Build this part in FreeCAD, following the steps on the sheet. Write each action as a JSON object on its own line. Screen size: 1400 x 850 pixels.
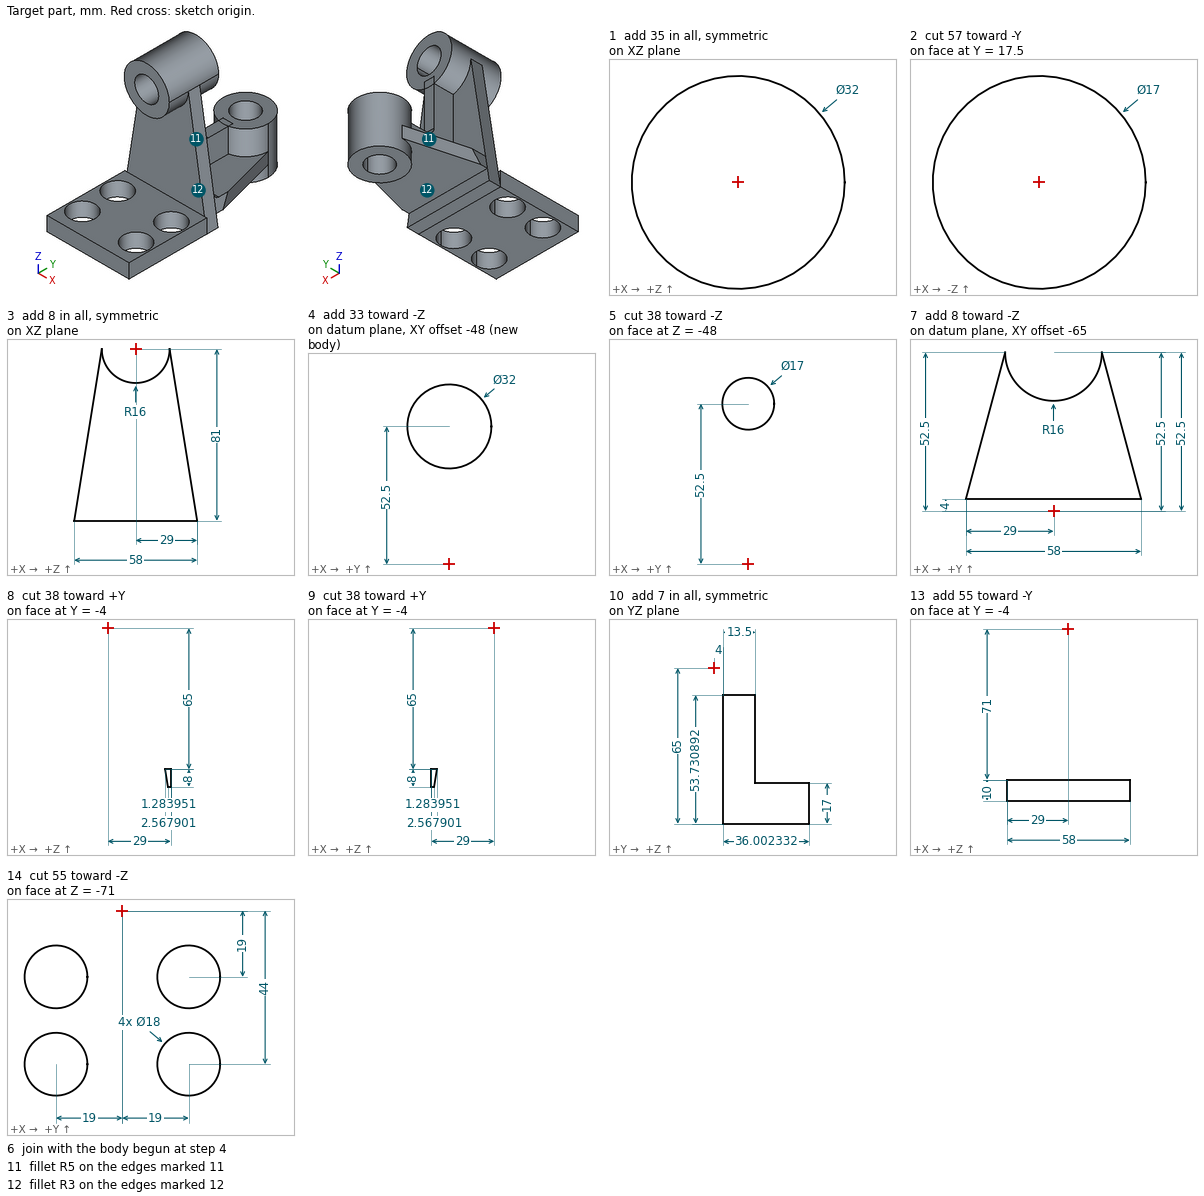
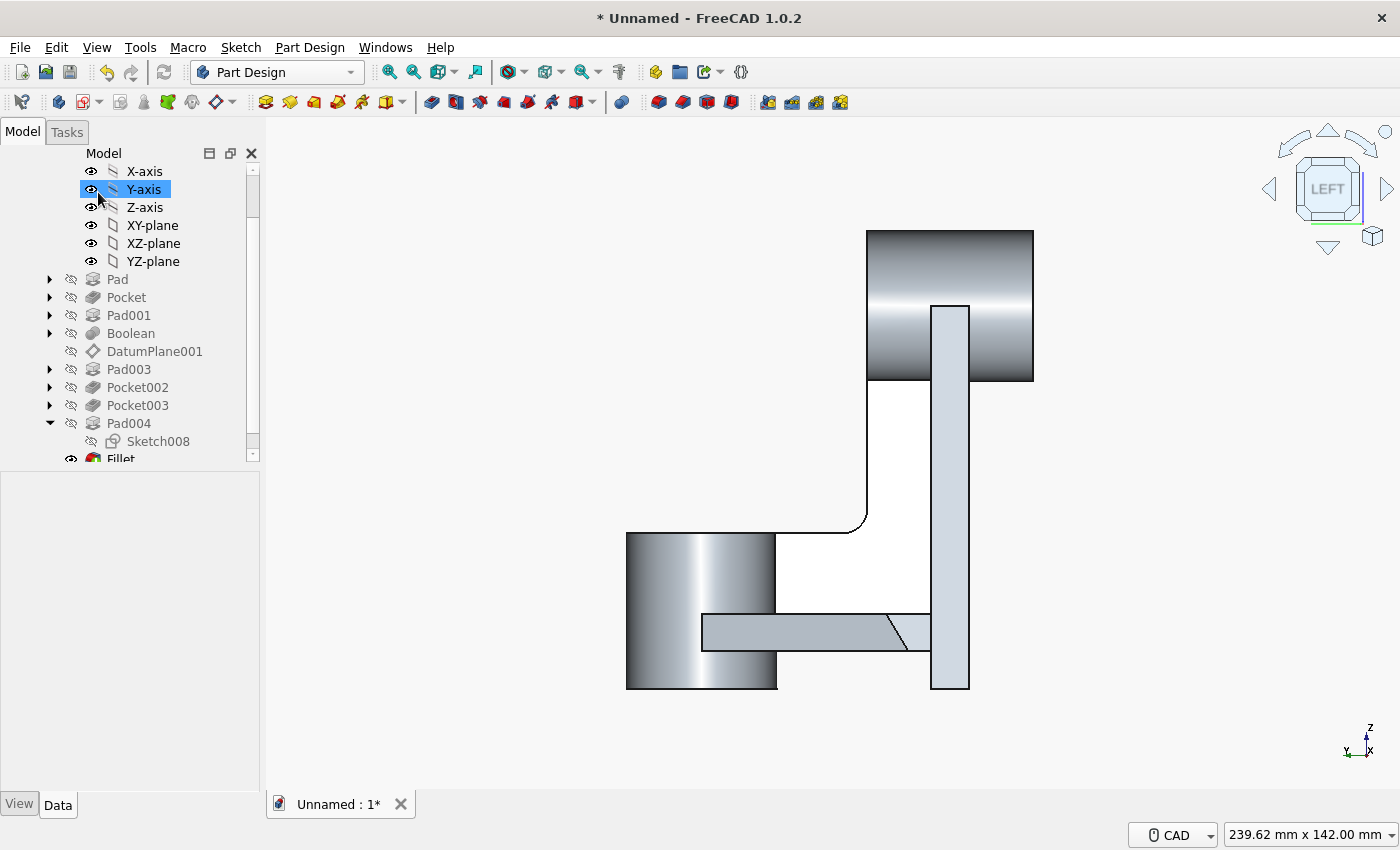
{"action": "key", "text": "v 3"}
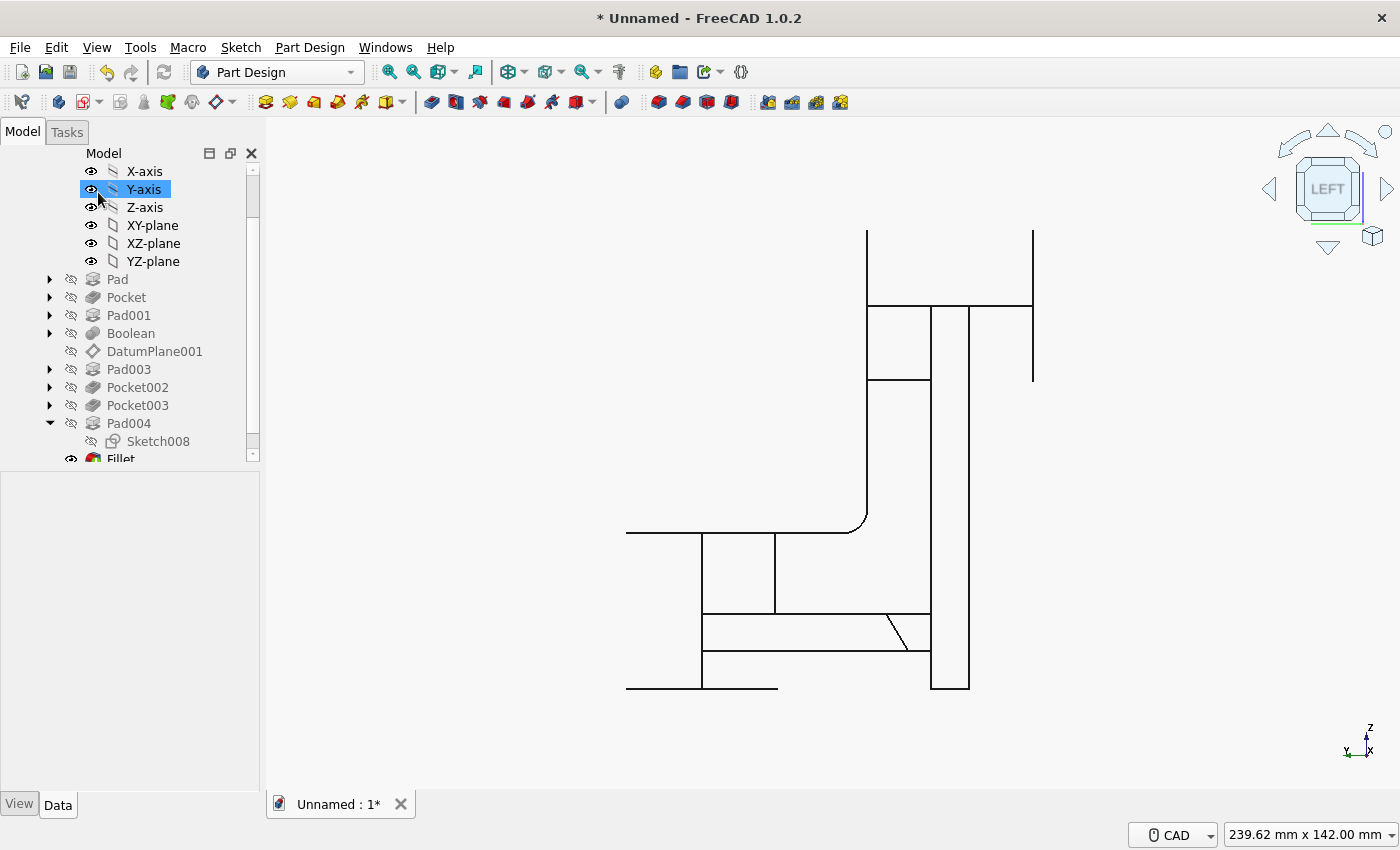
{"action": "key", "text": "0"}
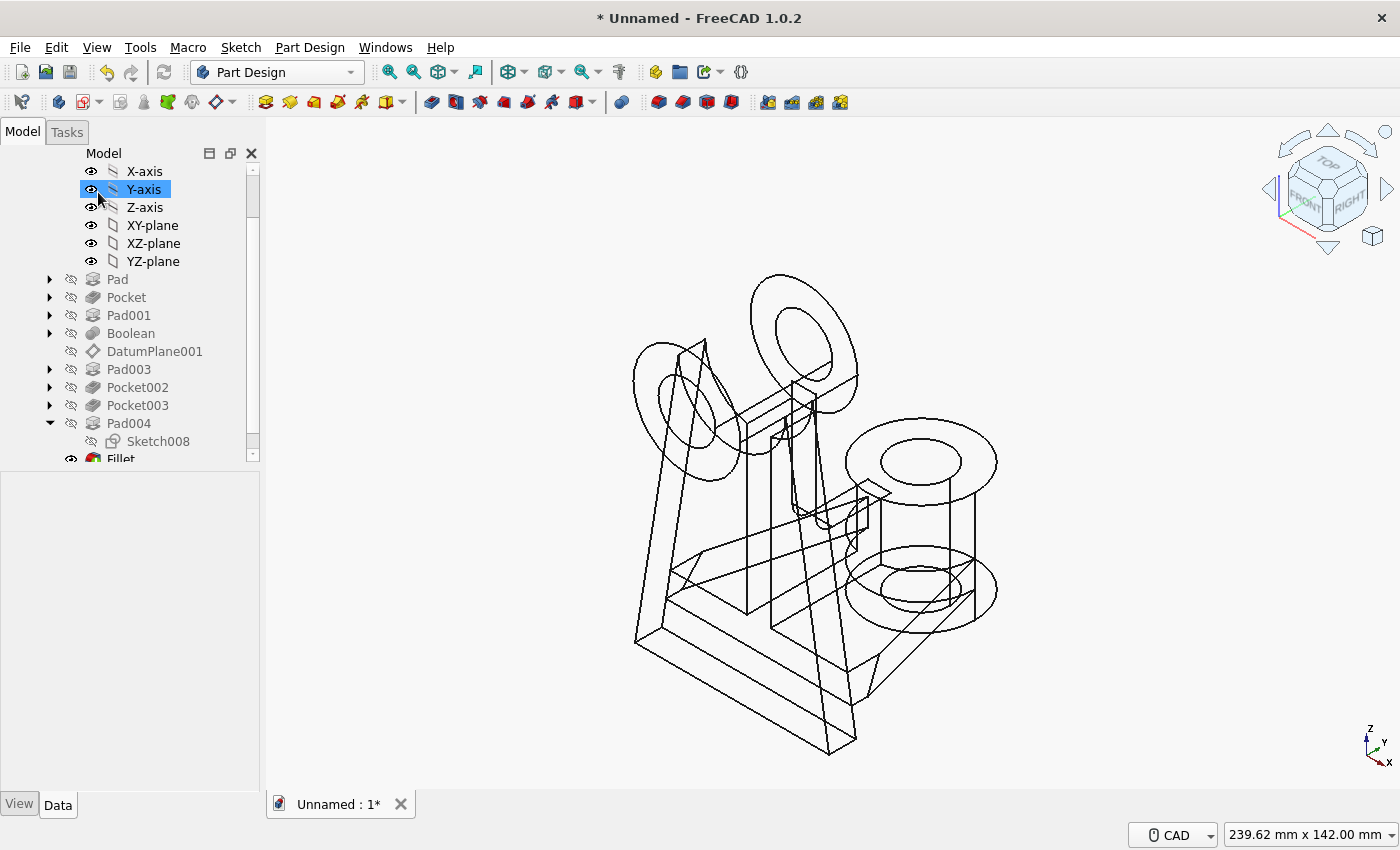
{"action": "left_click", "coordinate": [809, 649]}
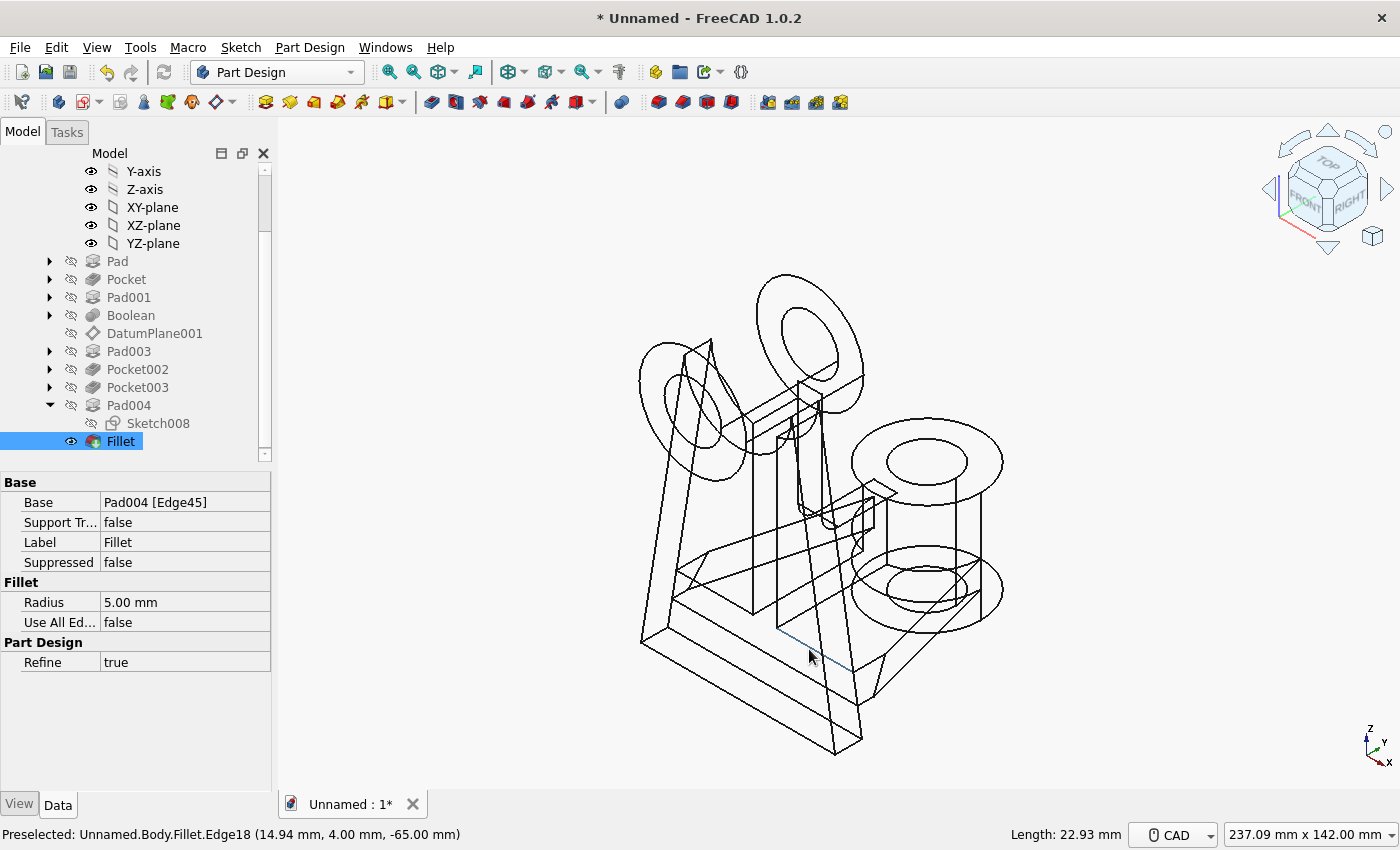
{"action": "key", "text": "v 1"}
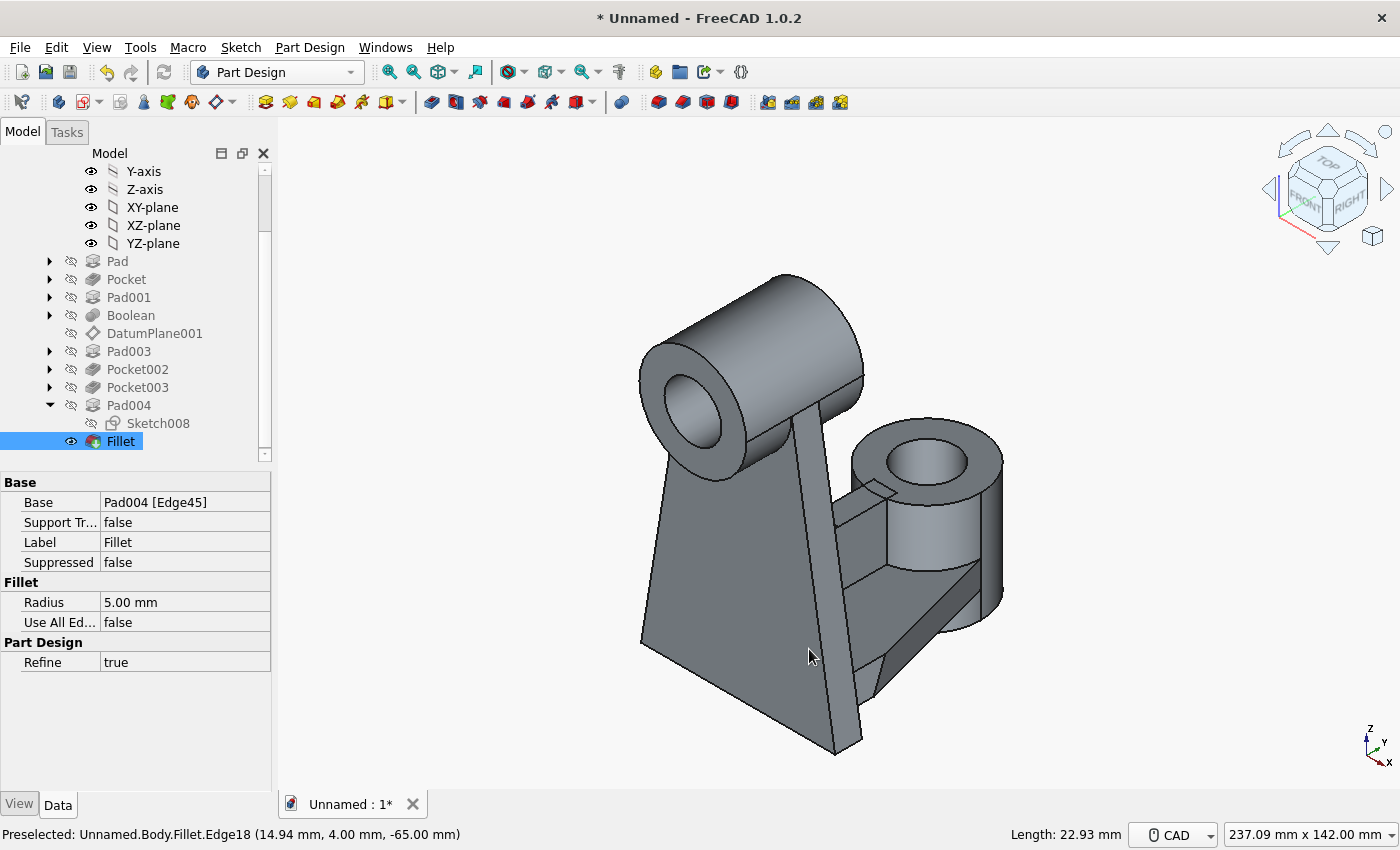
{"action": "left_click", "coordinate": [660, 102]}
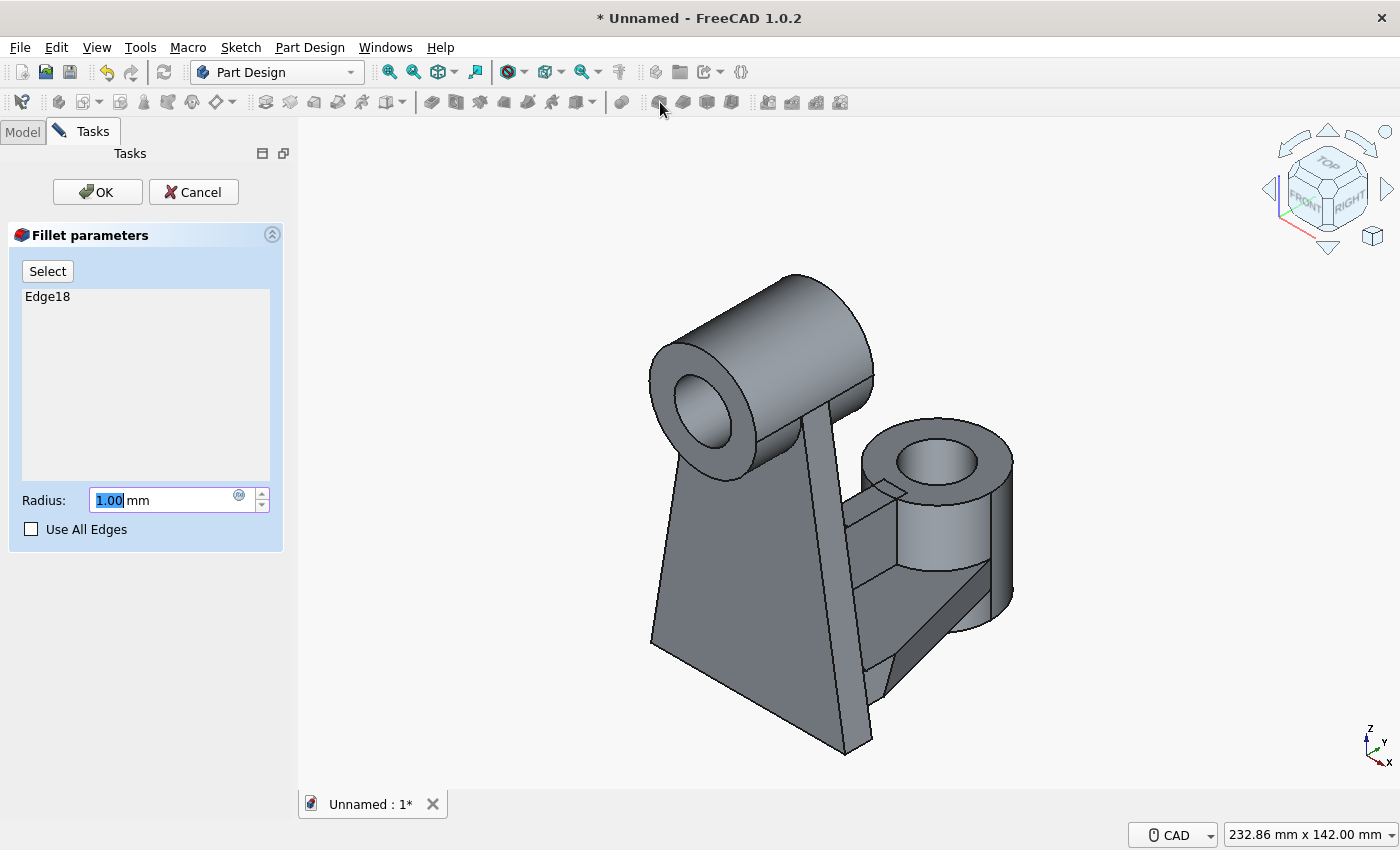
{"action": "type", "text": "3"}
{"action": "key", "text": "Tab"}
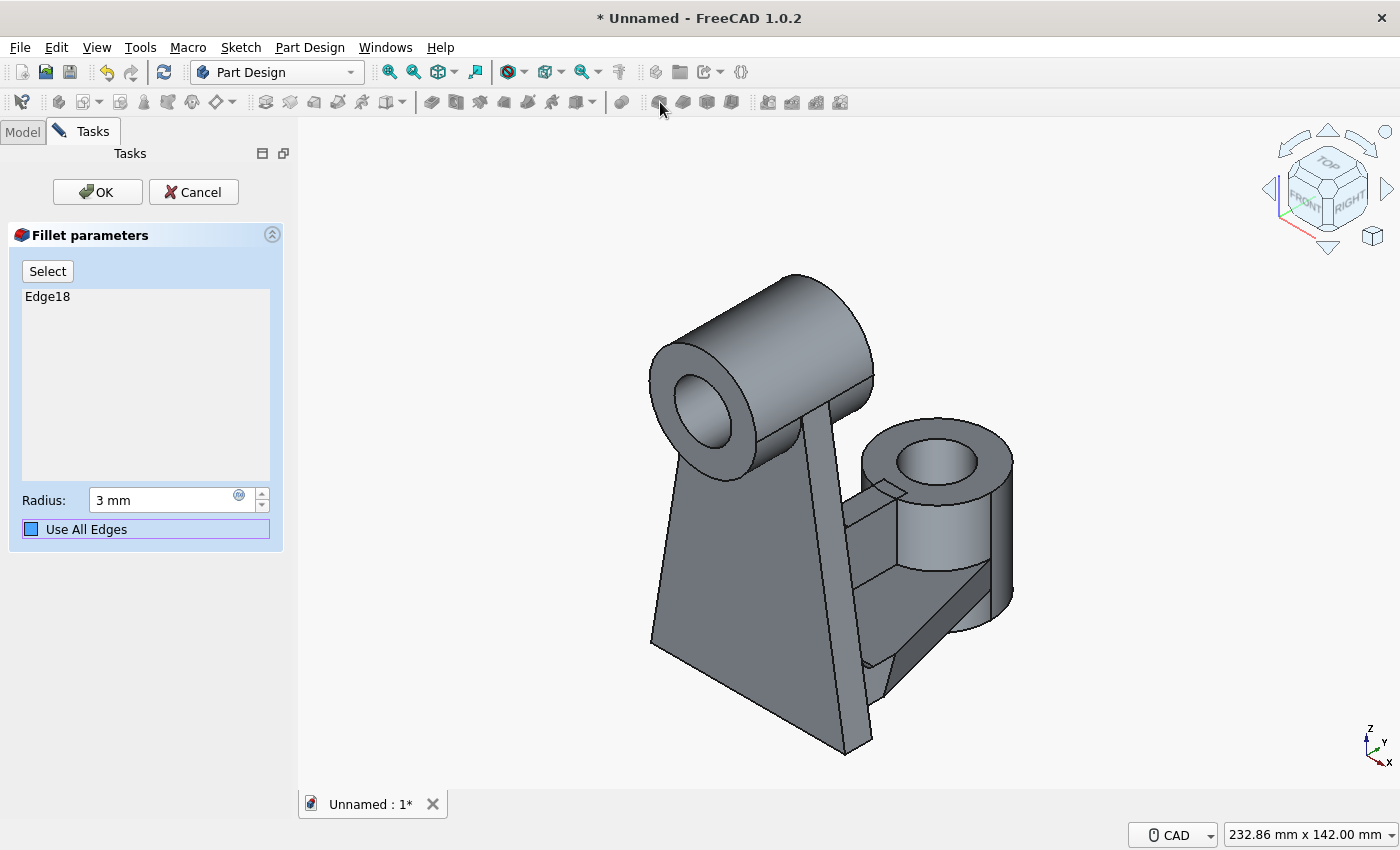
{"action": "left_click", "coordinate": [98, 192]}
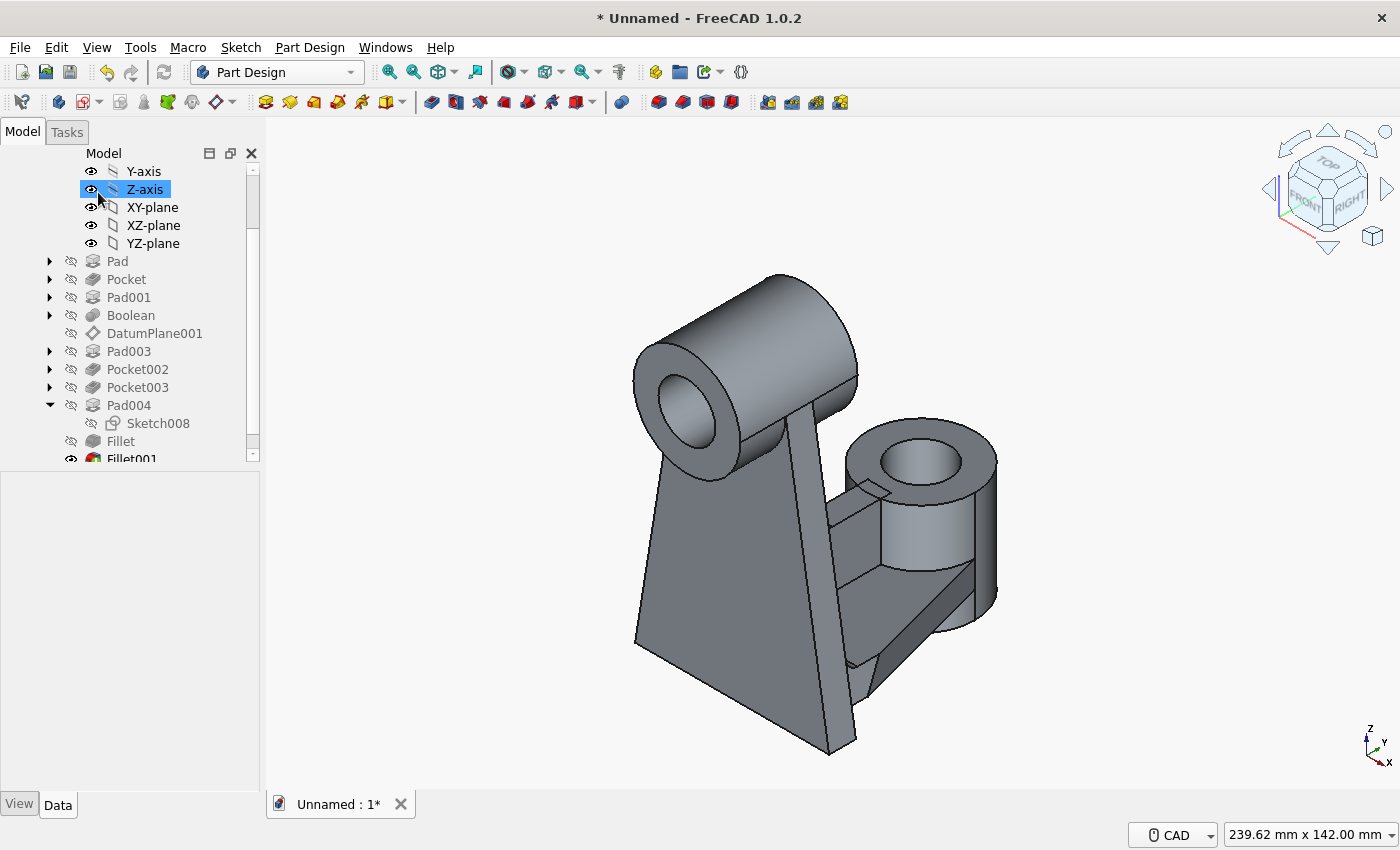
{"action": "left_click", "coordinate": [732, 586]}